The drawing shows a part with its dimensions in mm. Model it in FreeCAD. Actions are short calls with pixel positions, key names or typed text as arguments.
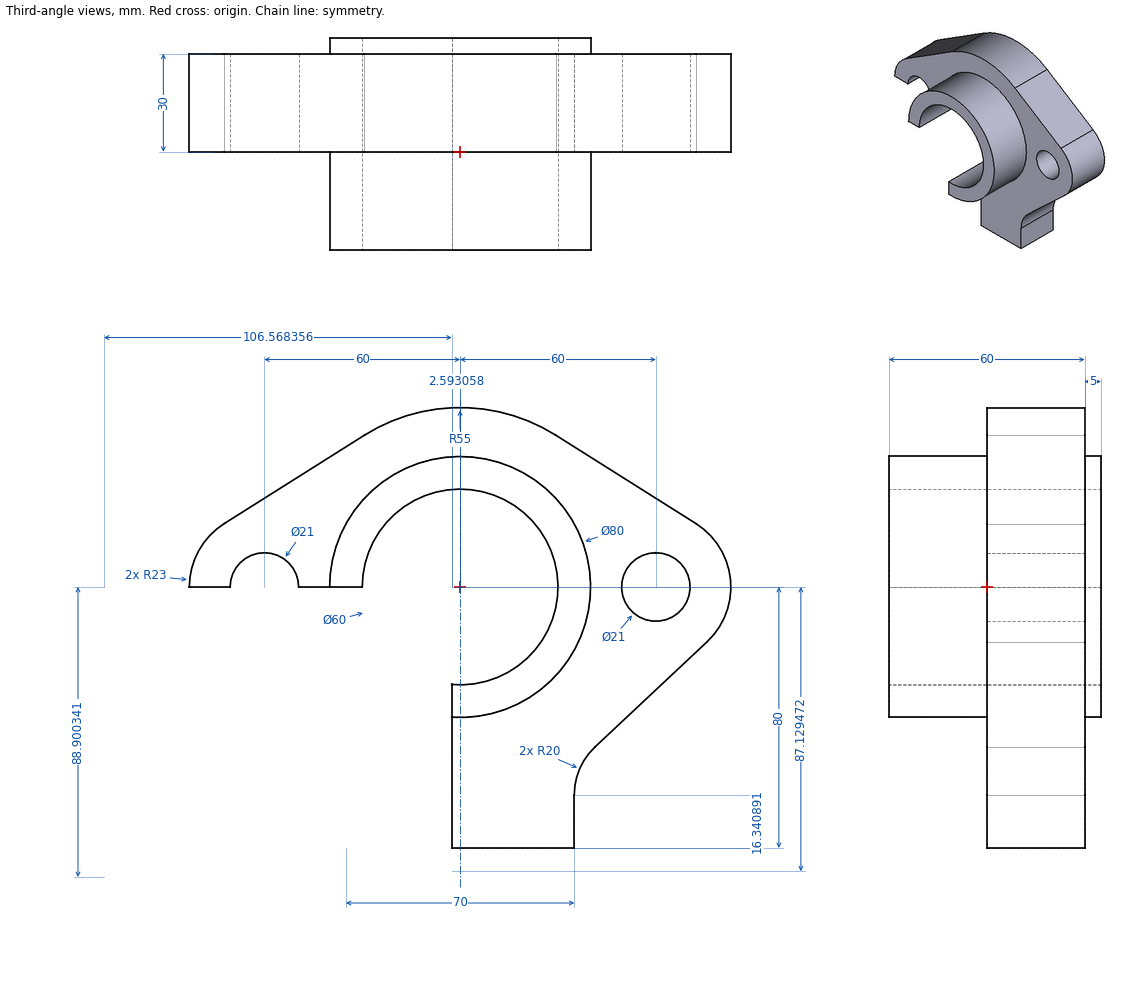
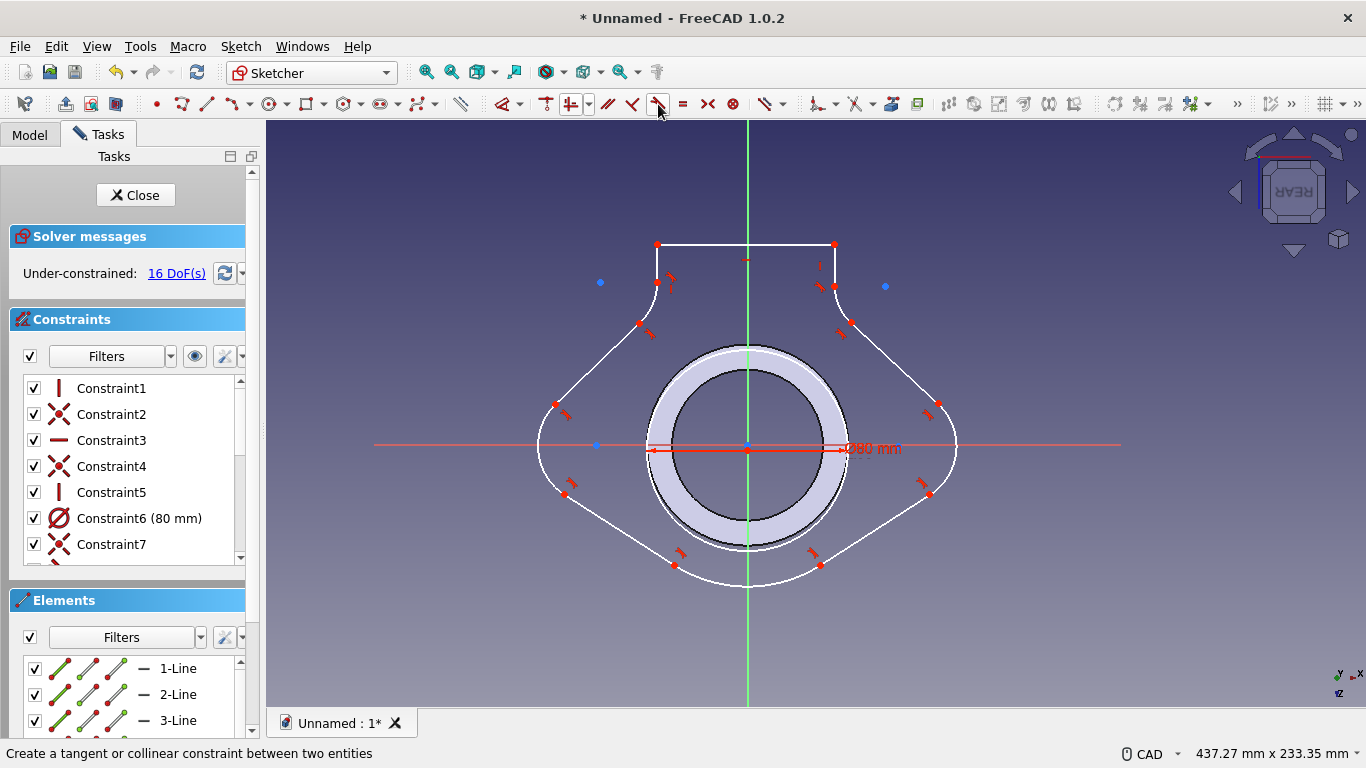
drag(737, 435, 758, 461)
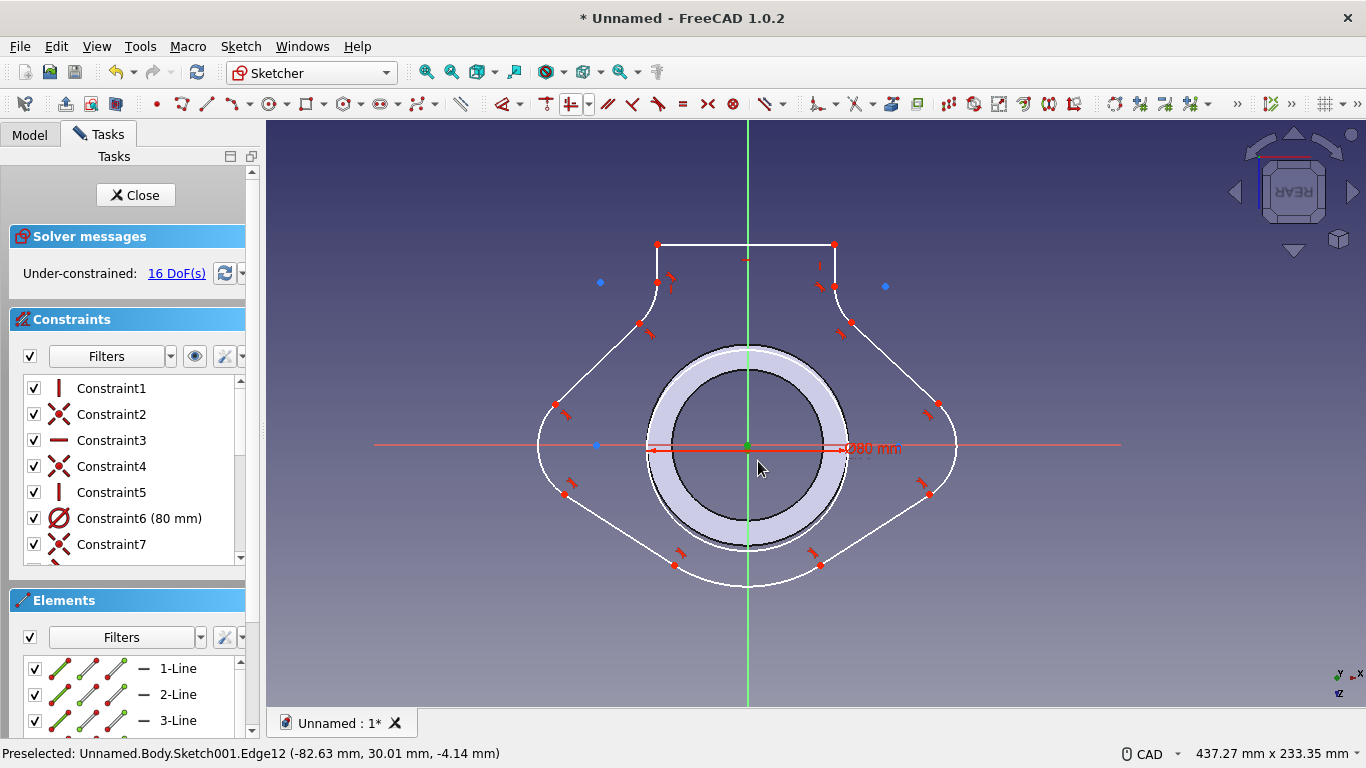
click(546, 104)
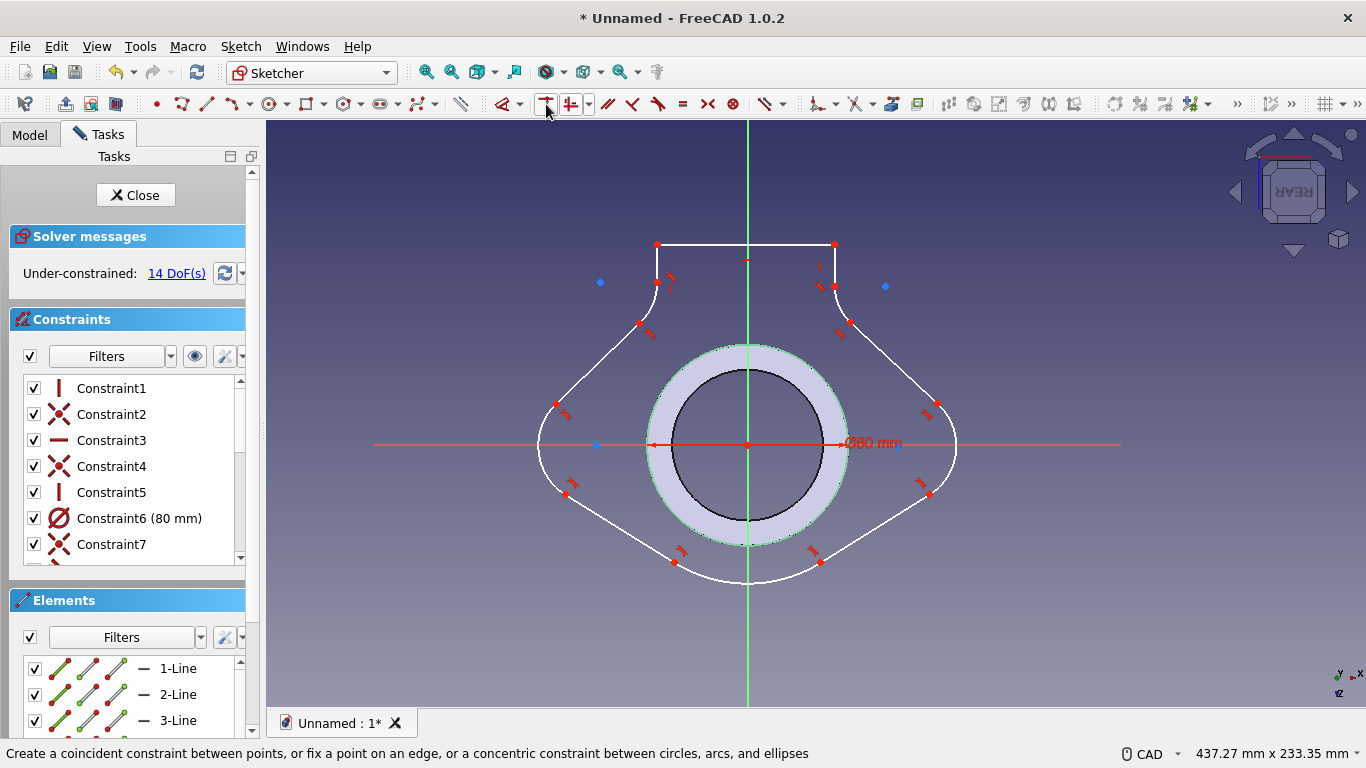
click(836, 298)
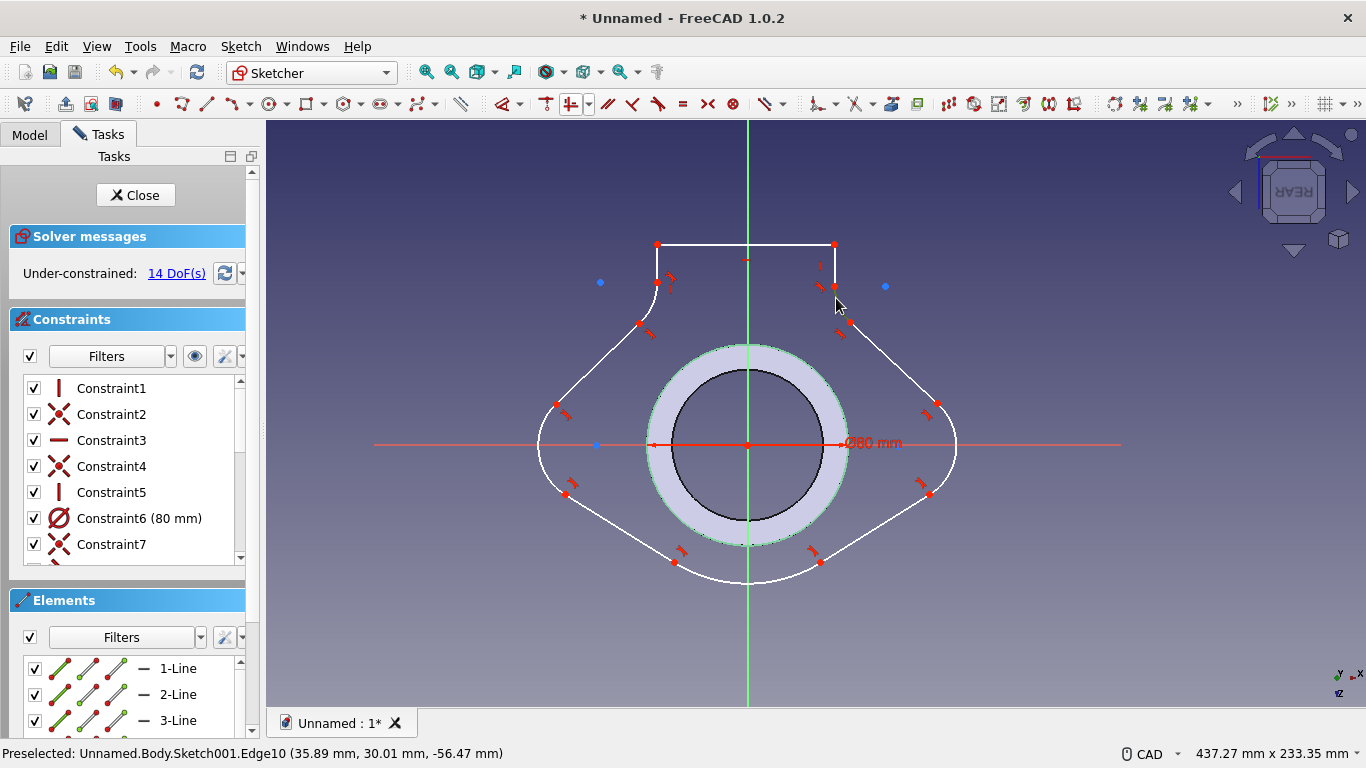
click(649, 312)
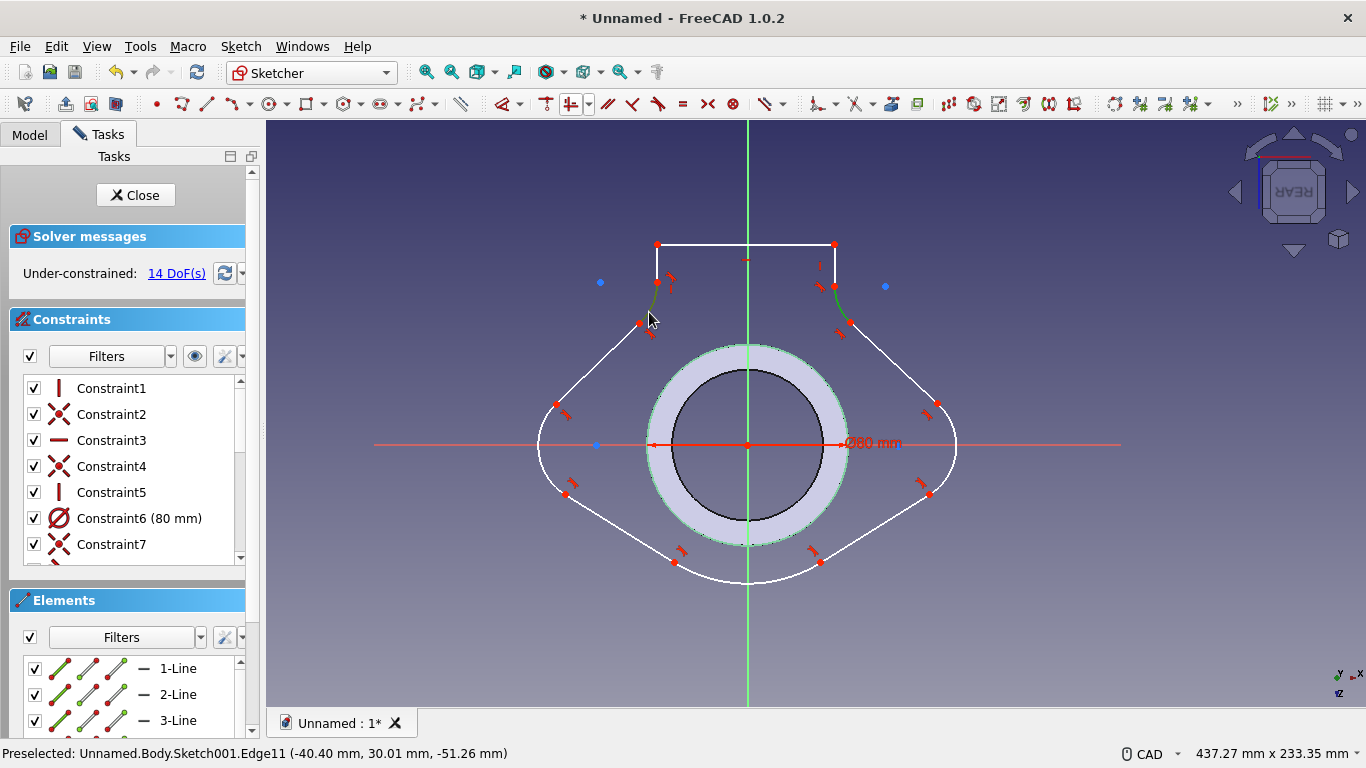
click(683, 104)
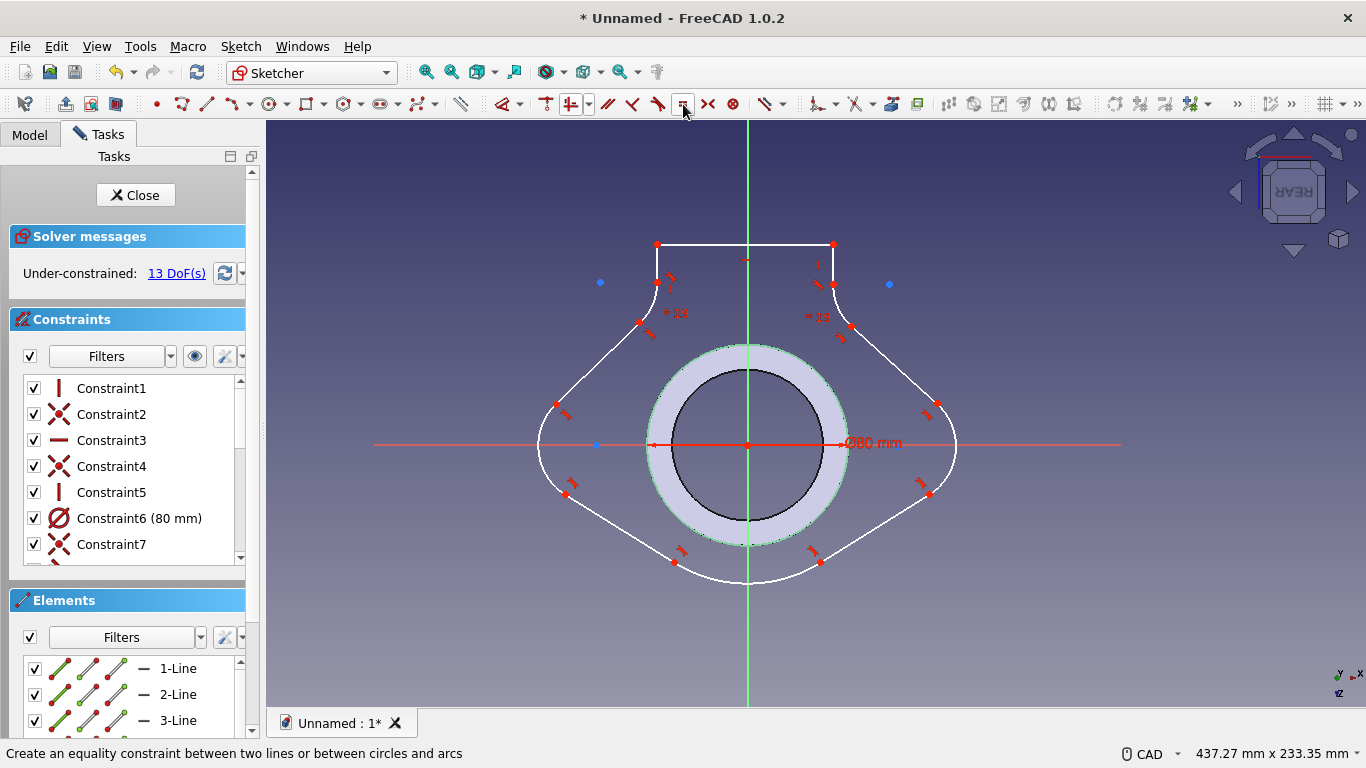
click(950, 472)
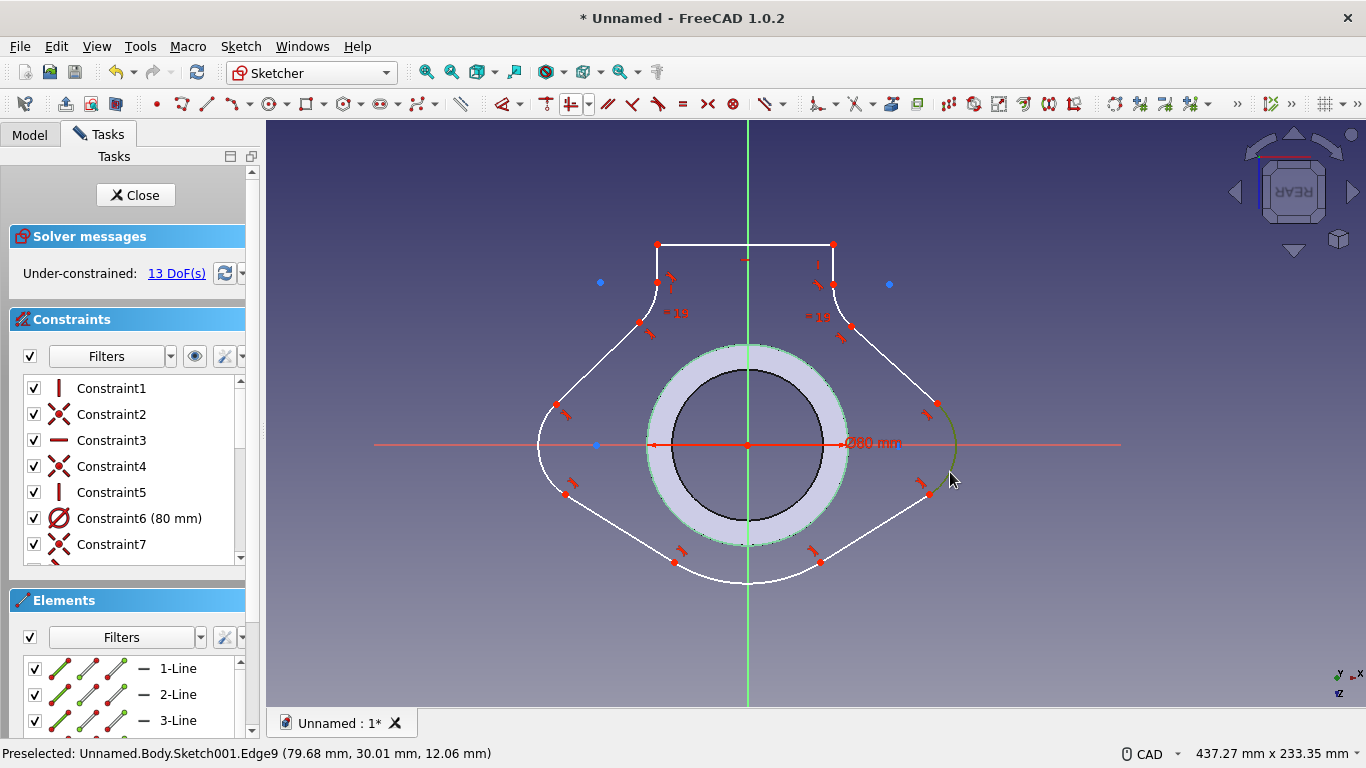
click(540, 431)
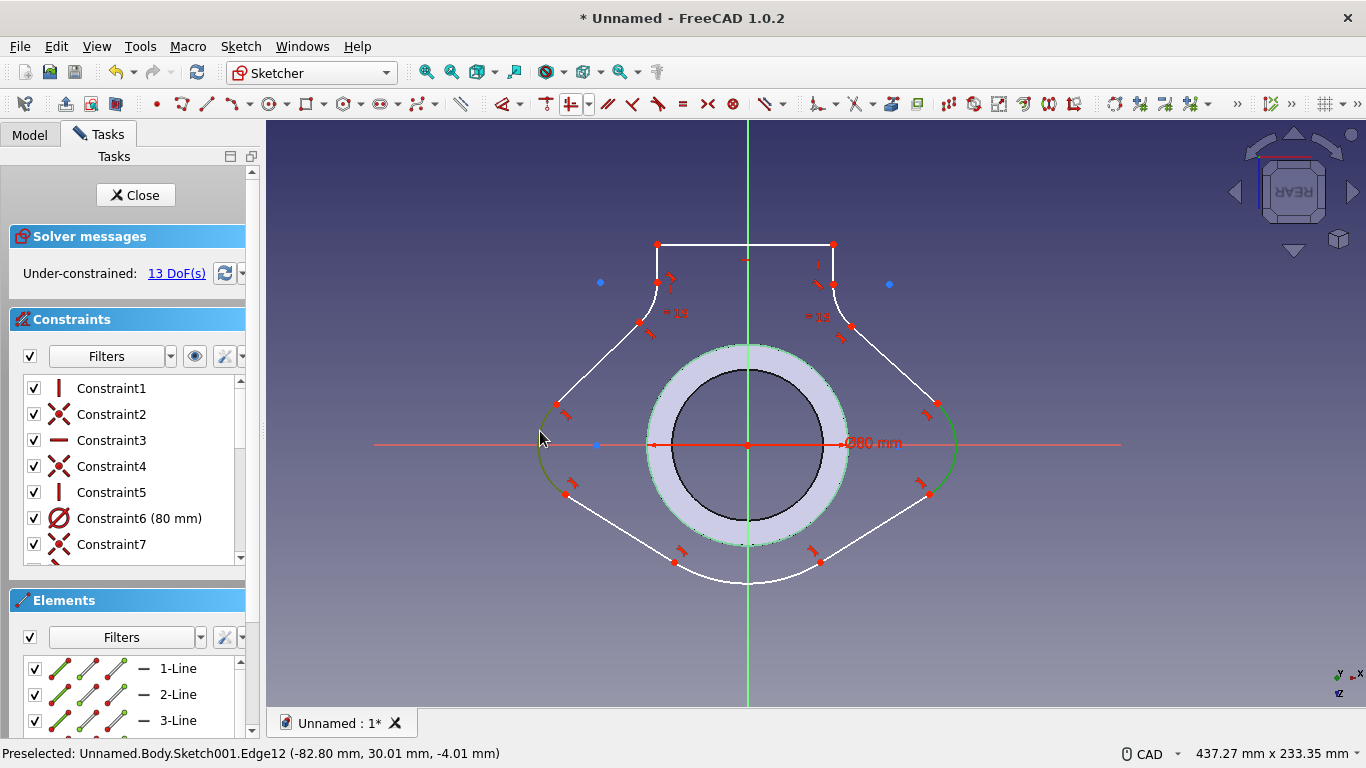
click(683, 104)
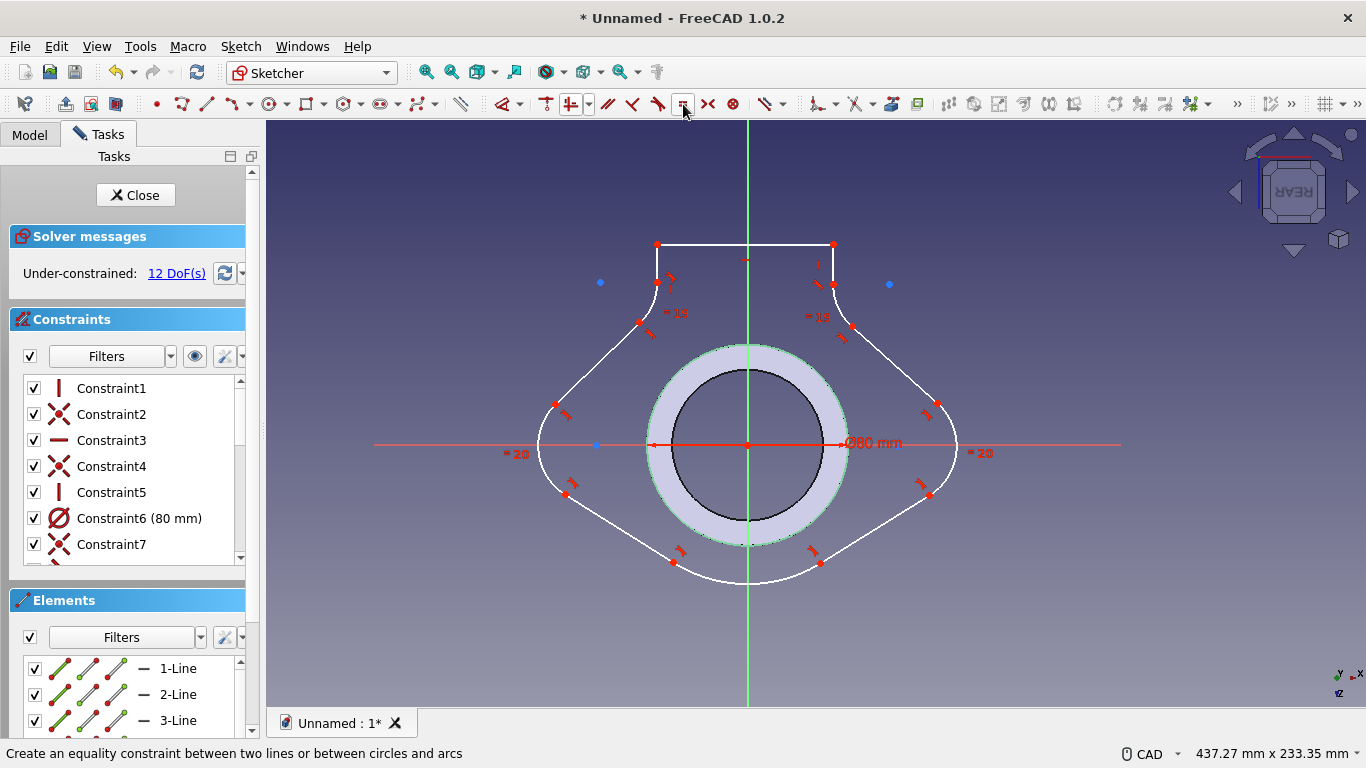
click(899, 446)